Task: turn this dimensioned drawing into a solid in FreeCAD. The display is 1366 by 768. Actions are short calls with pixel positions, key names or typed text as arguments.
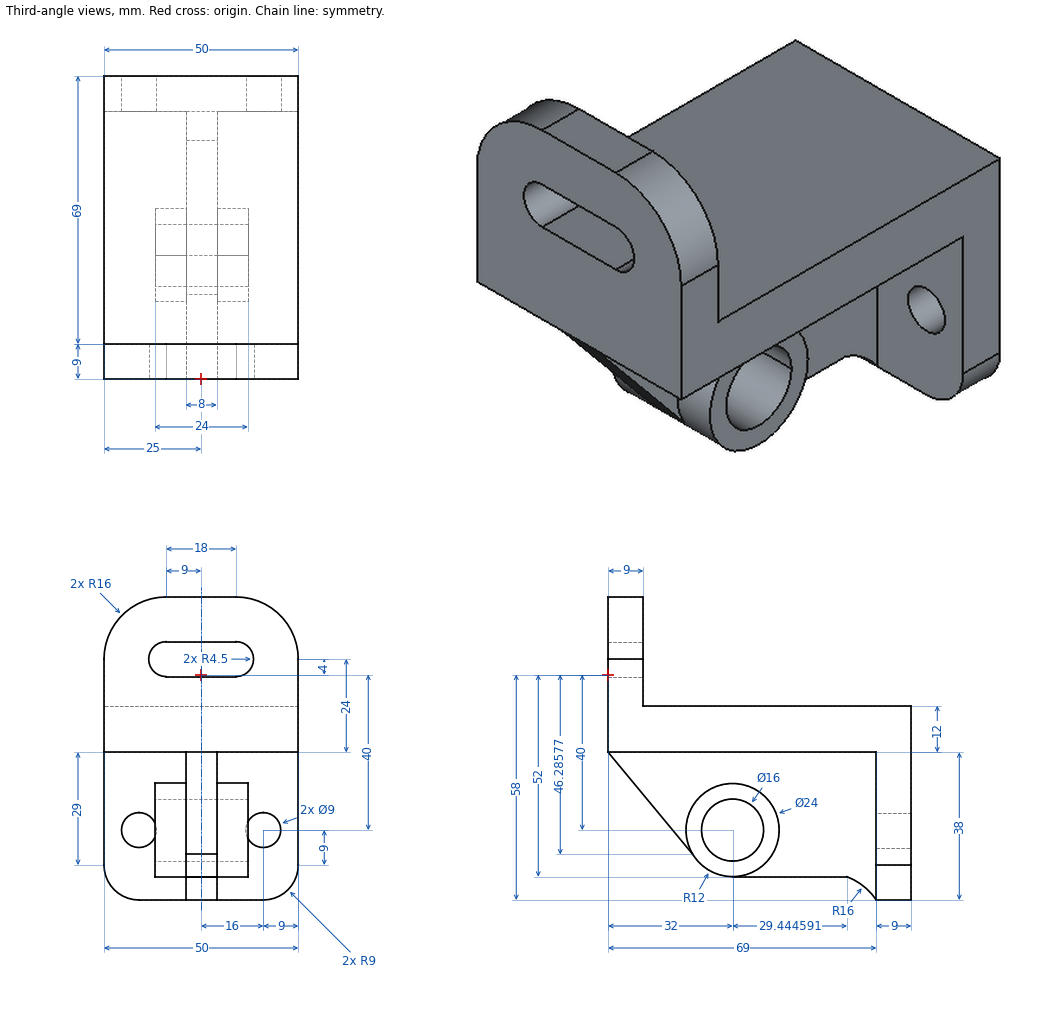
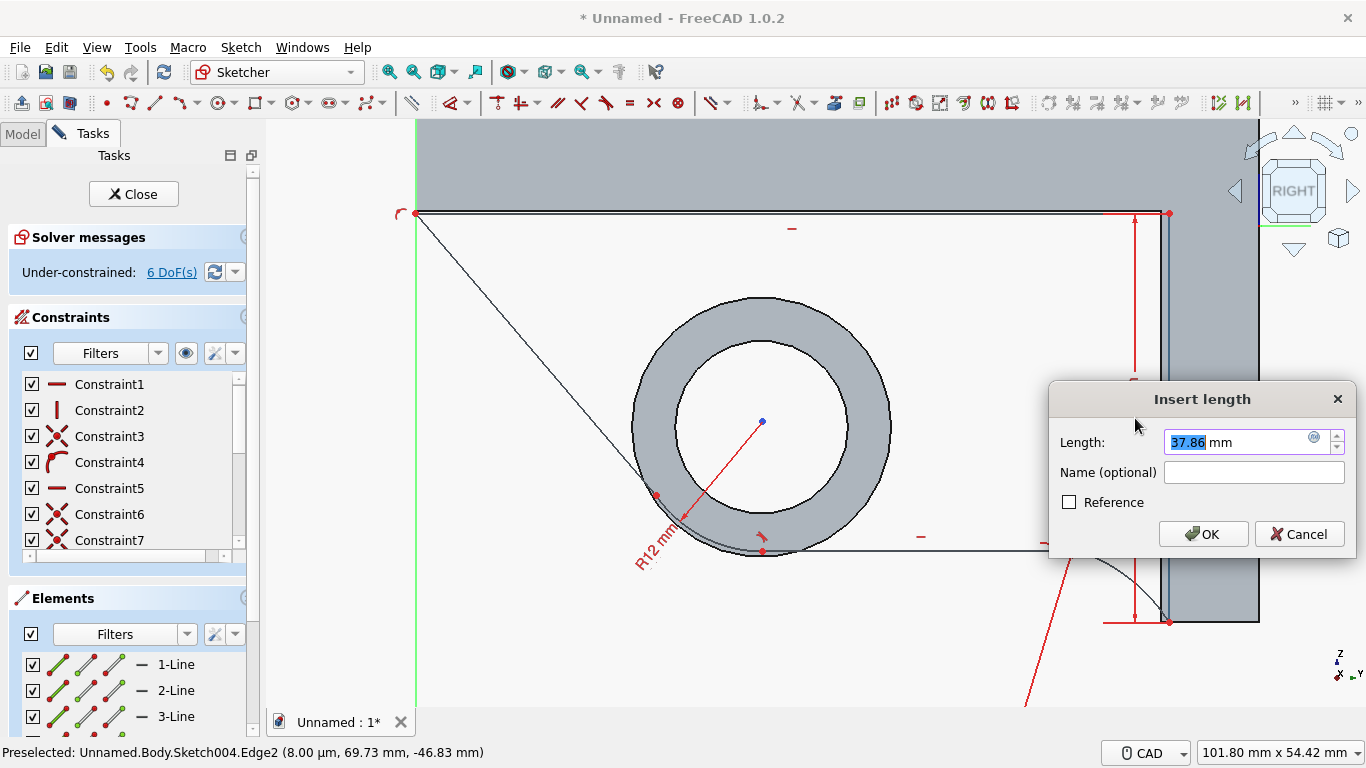
text(38)
key(Return)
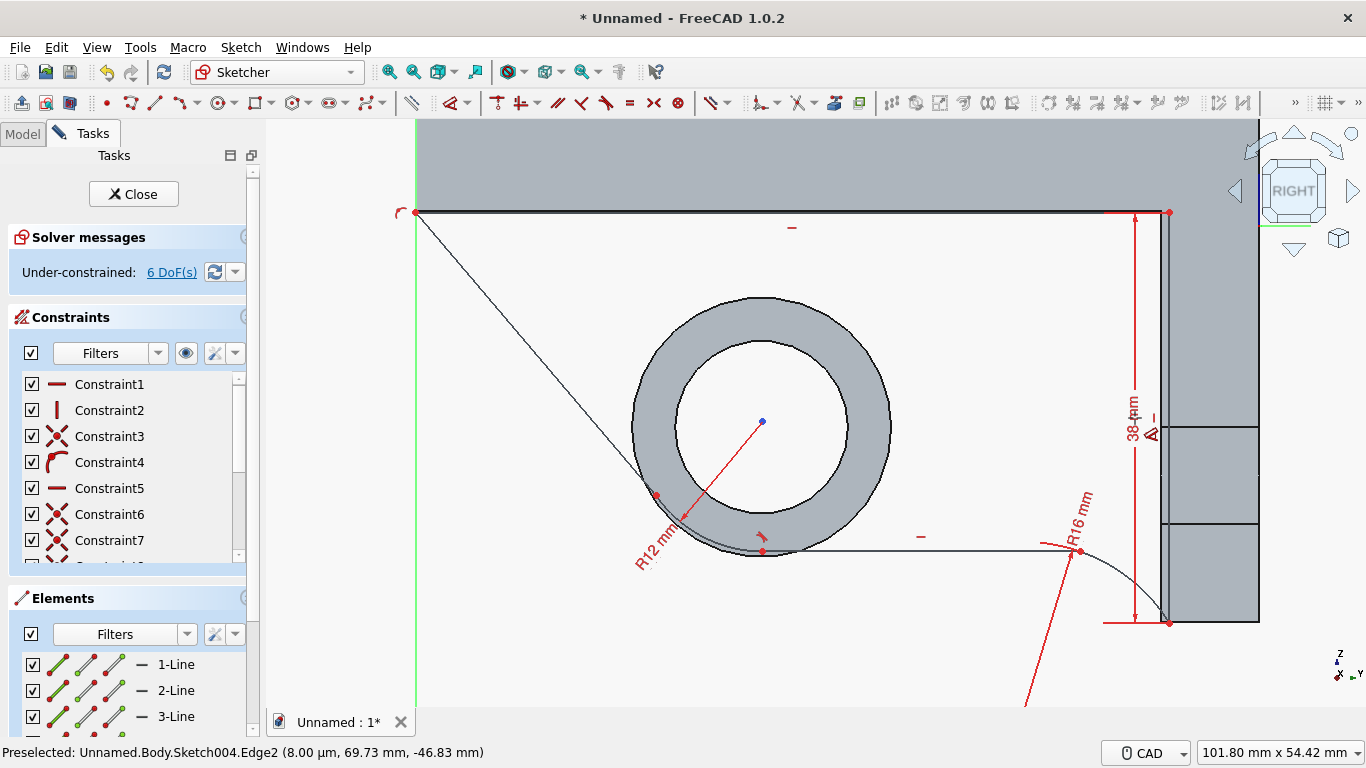
click(943, 212)
click(793, 178)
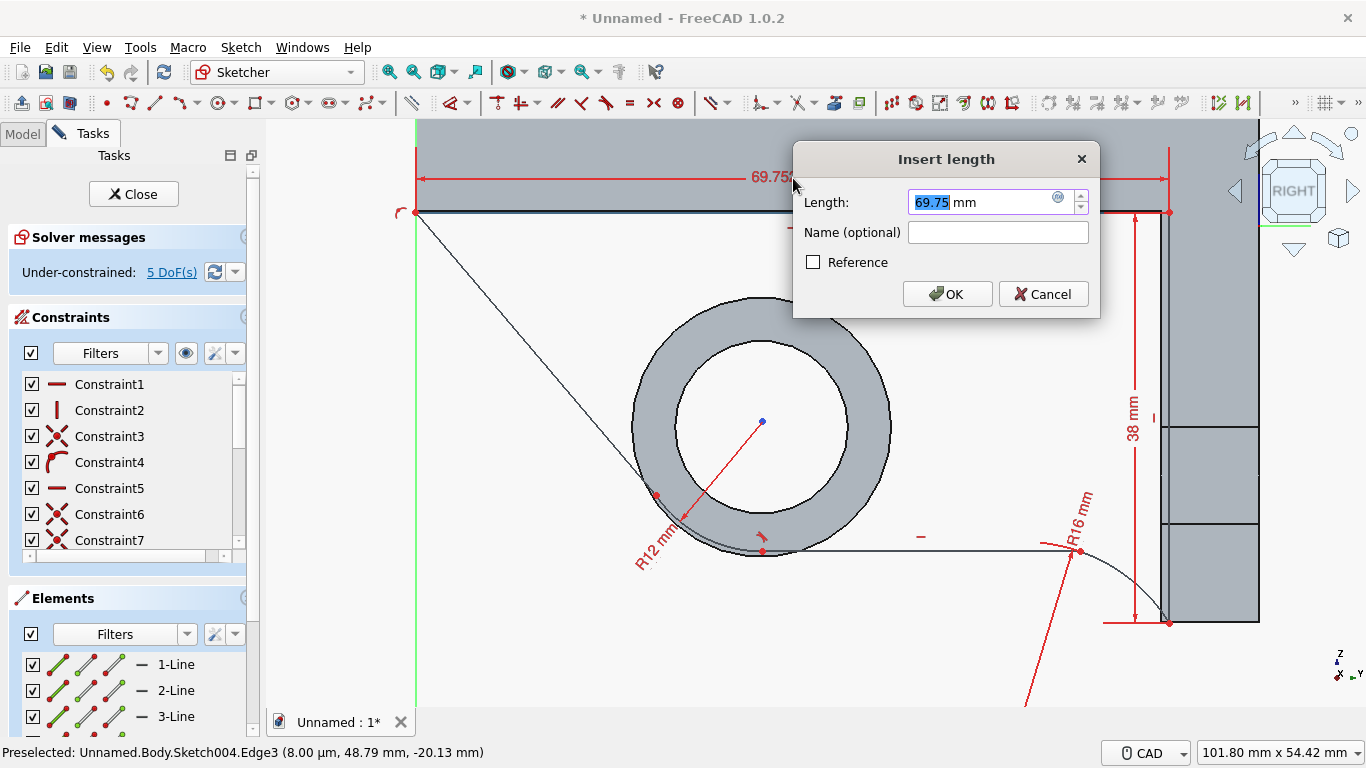
text(69)
key(Return)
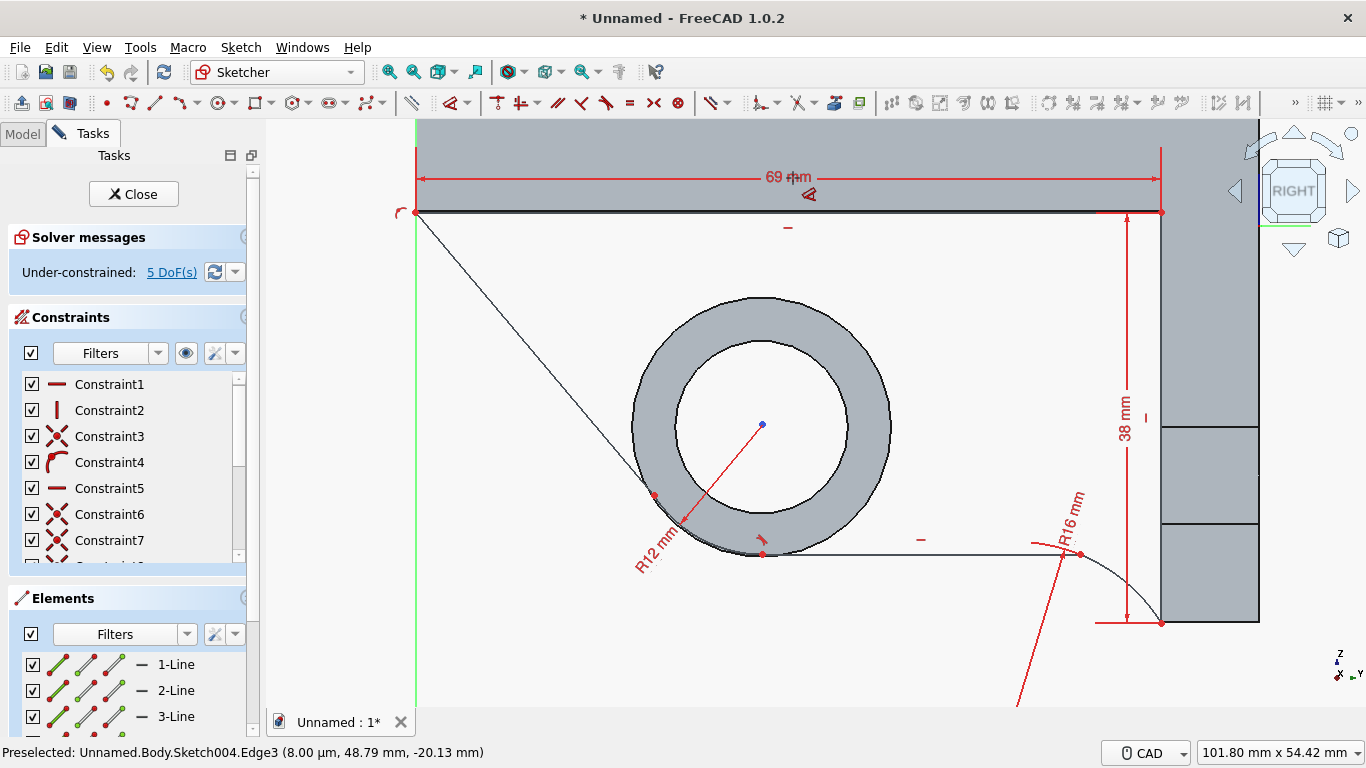
click(763, 555)
click(589, 589)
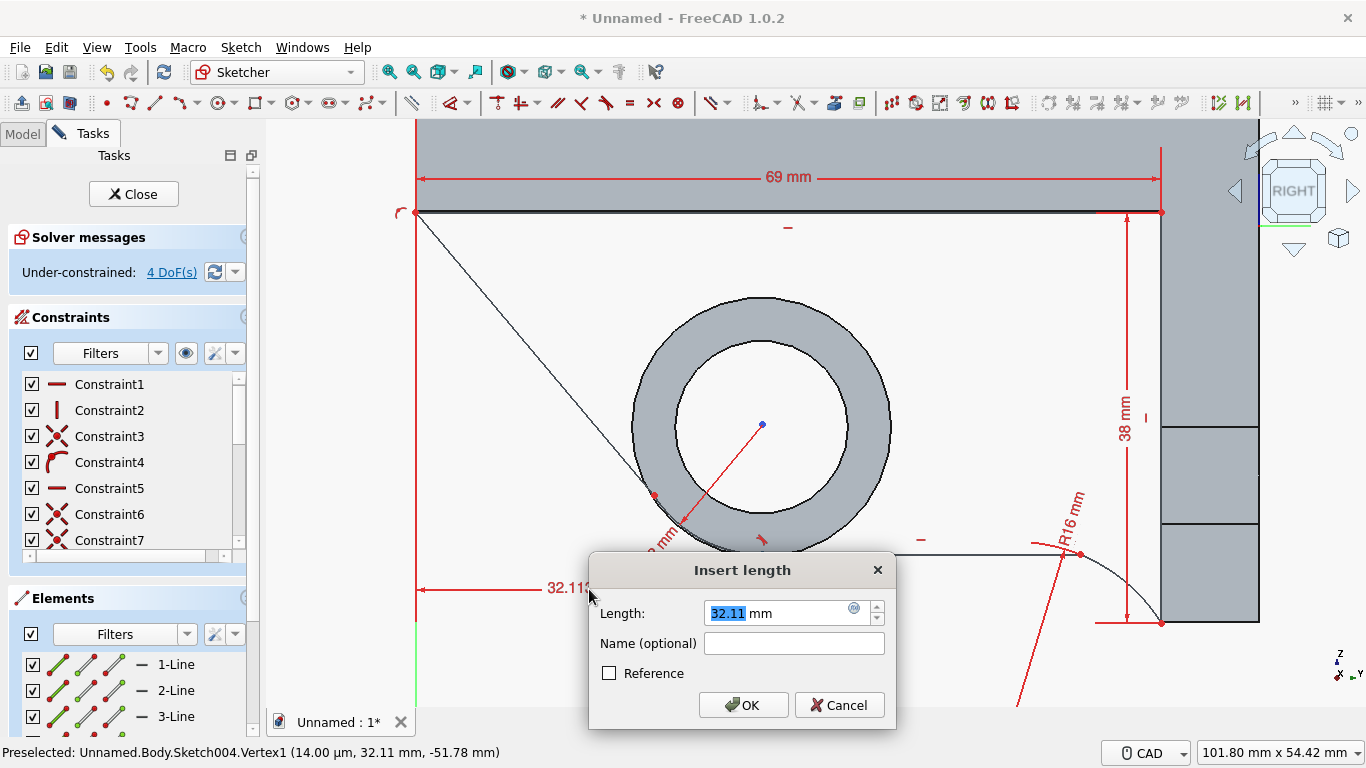
text(32)
key(Return)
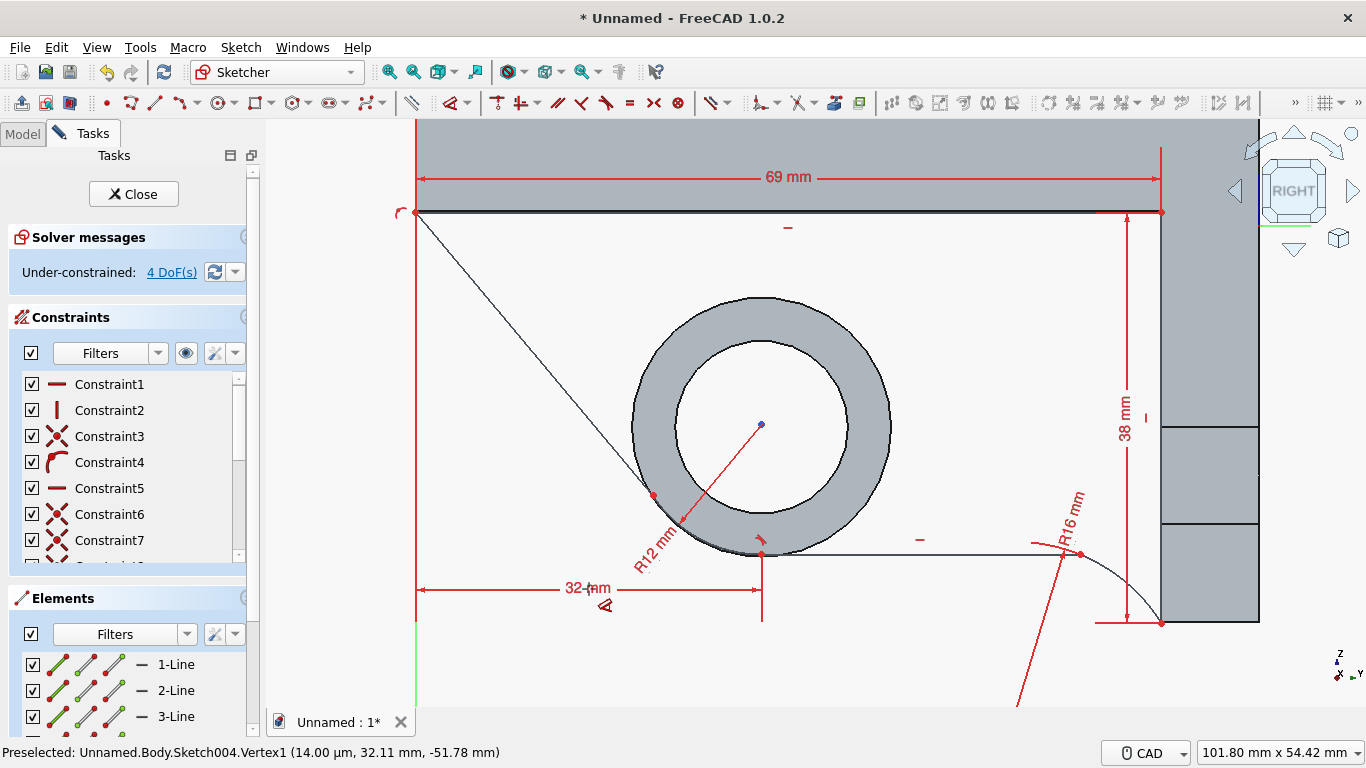
click(762, 555)
click(382, 351)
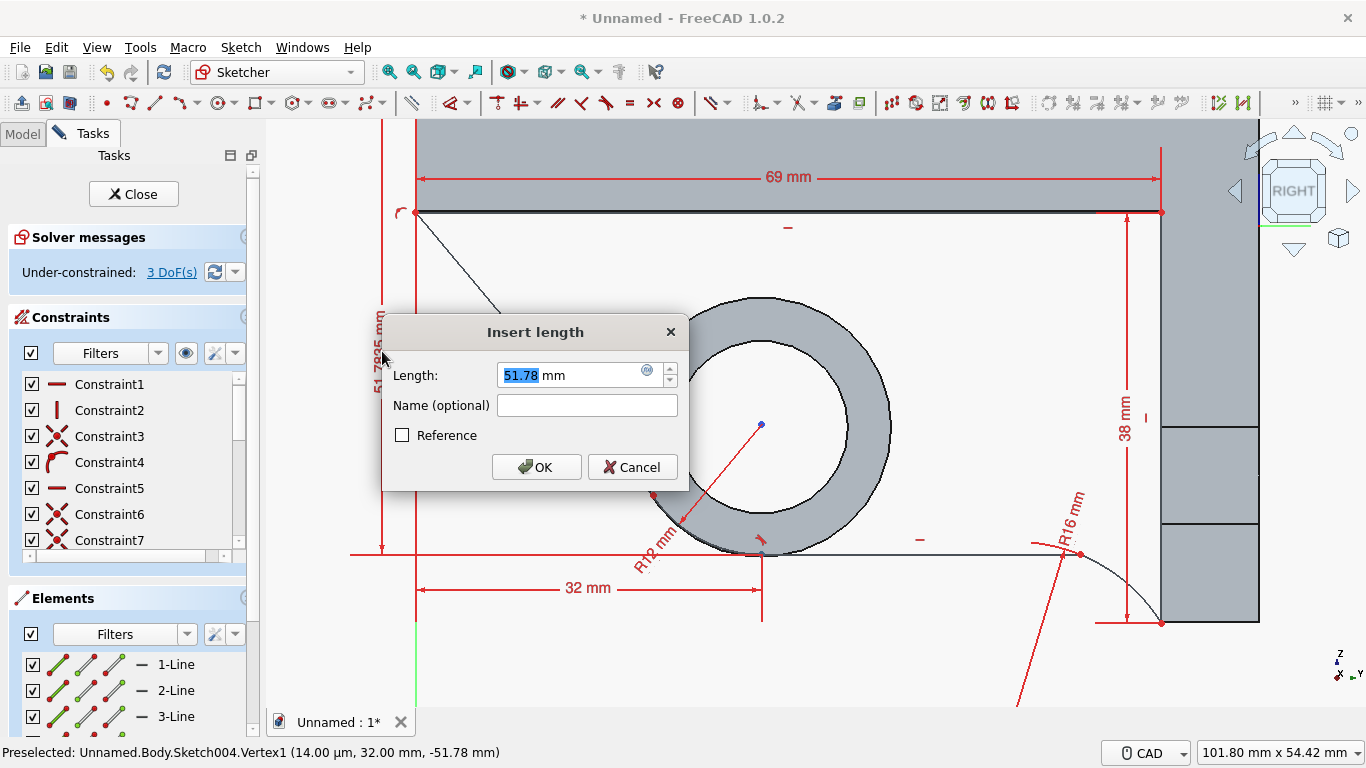
text(52)
key(Return)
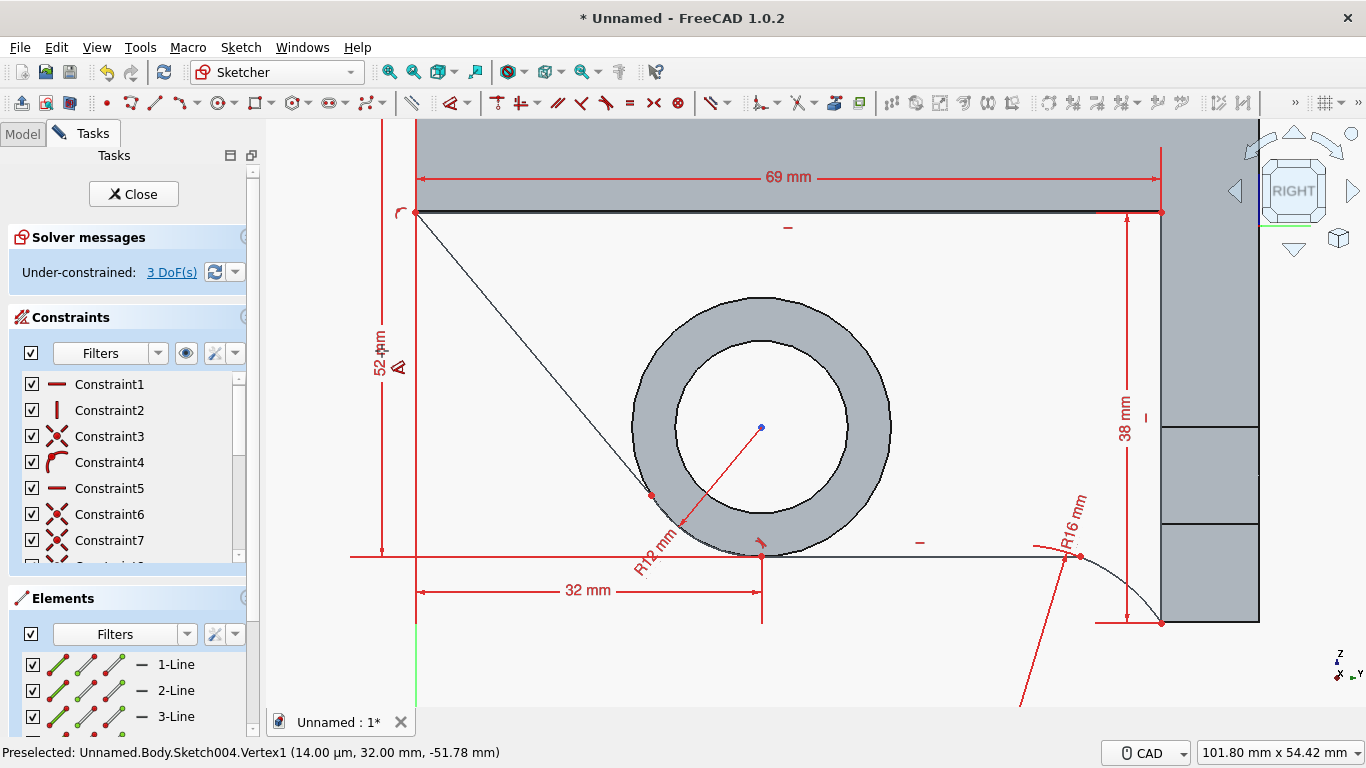
click(1161, 623)
click(1195, 385)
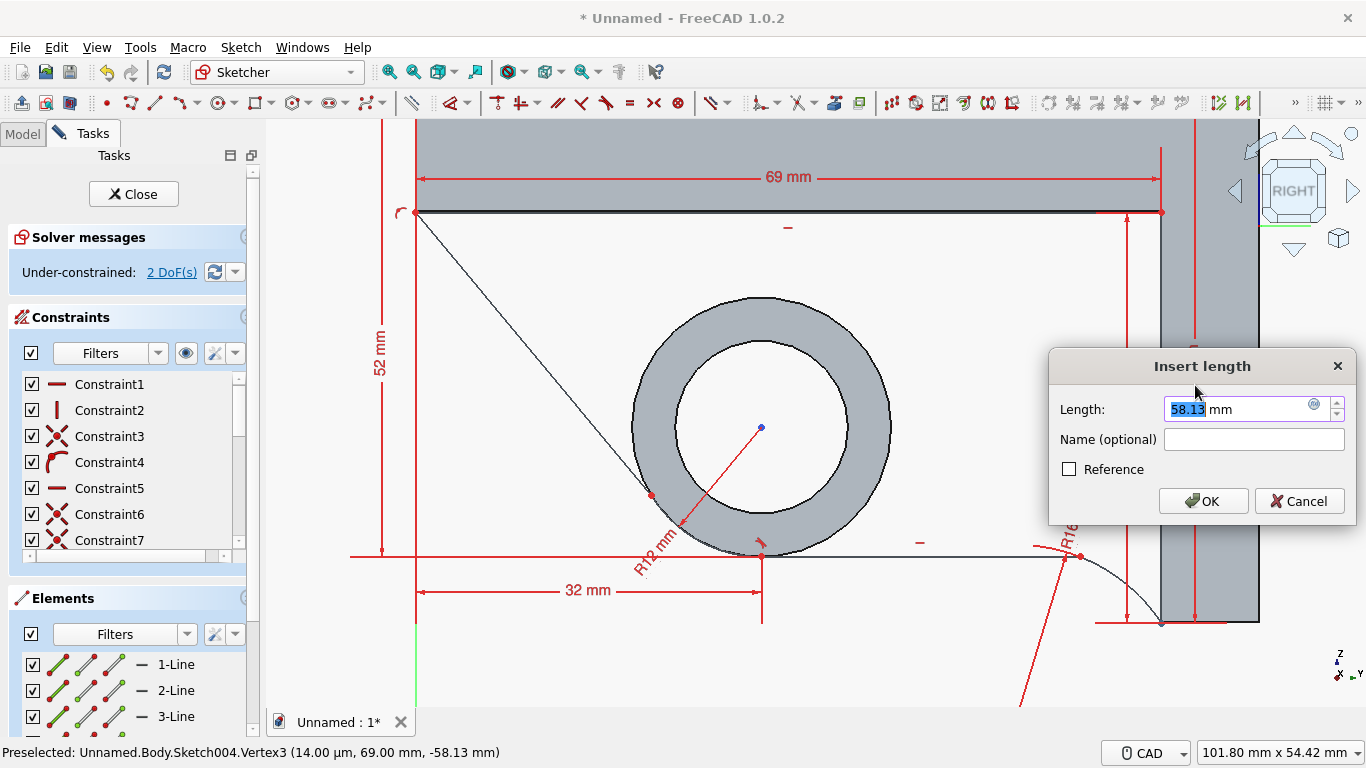
text(58)
key(Return)